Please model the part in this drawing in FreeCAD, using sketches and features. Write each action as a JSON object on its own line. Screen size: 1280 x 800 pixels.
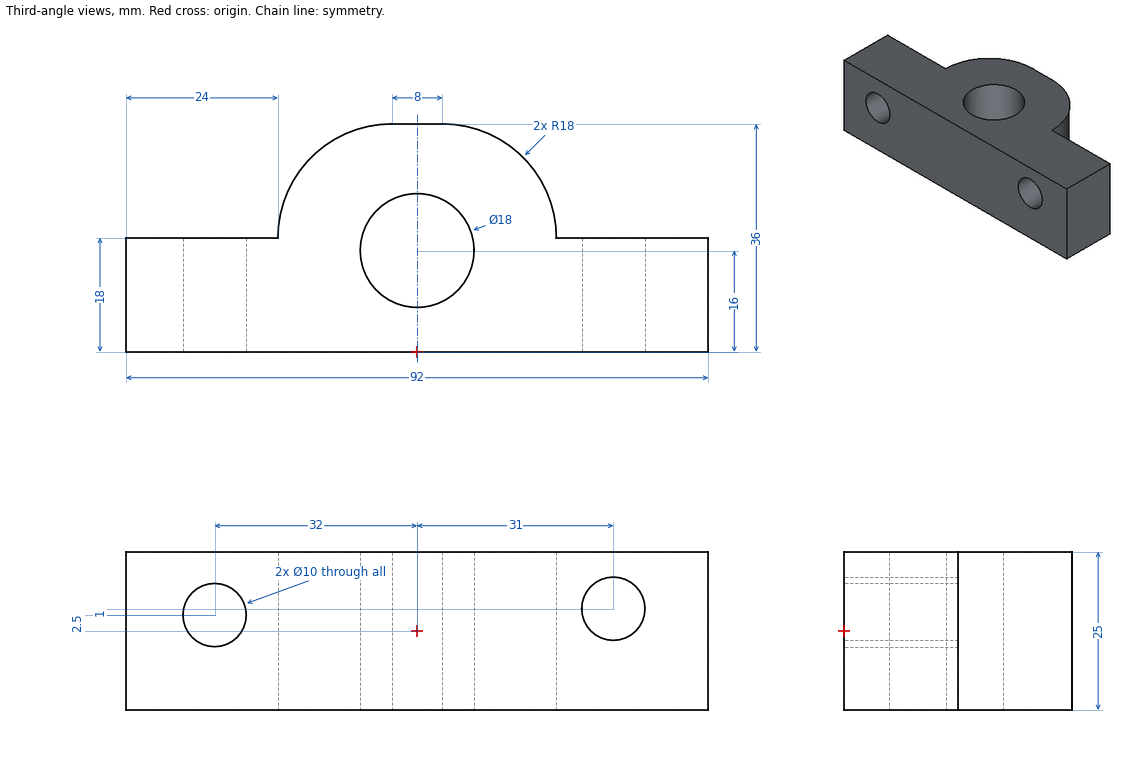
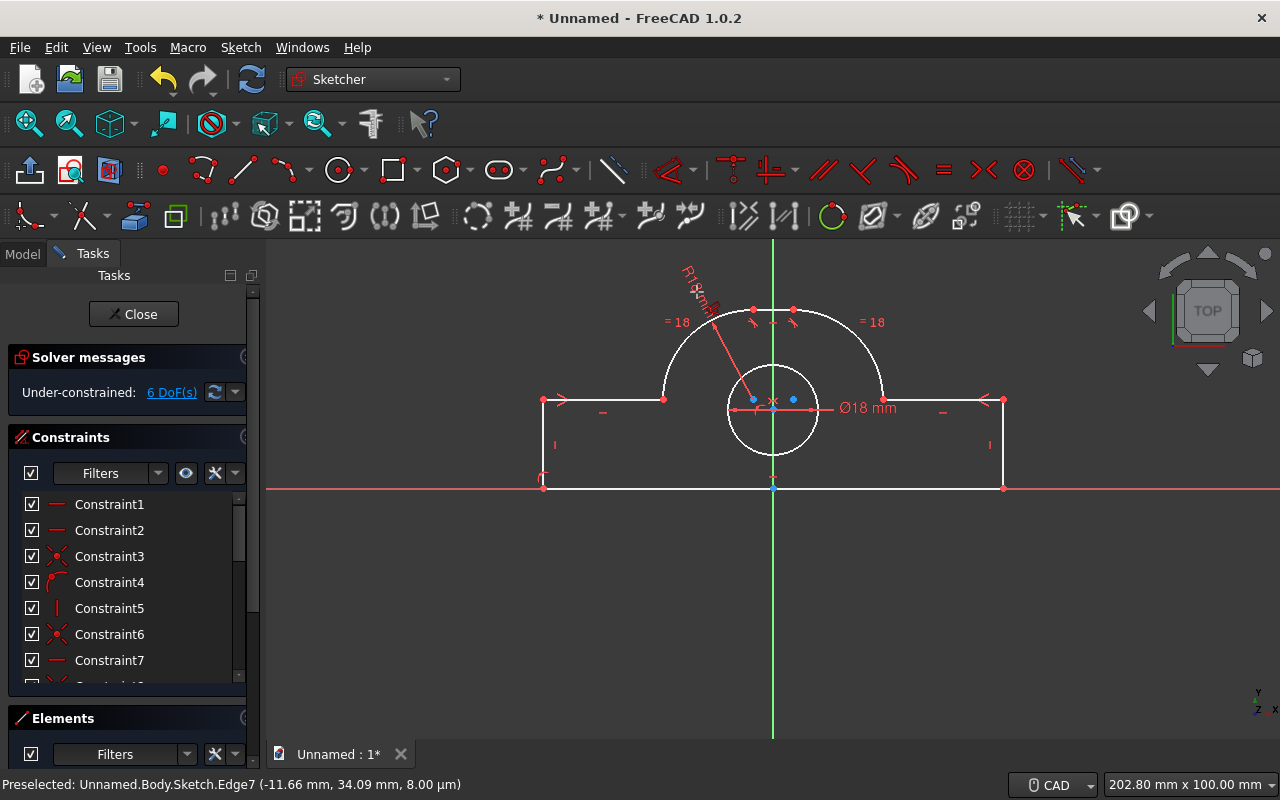
{"action": "left_click", "coordinate": [769, 310]}
{"action": "left_click", "coordinate": [787, 276]}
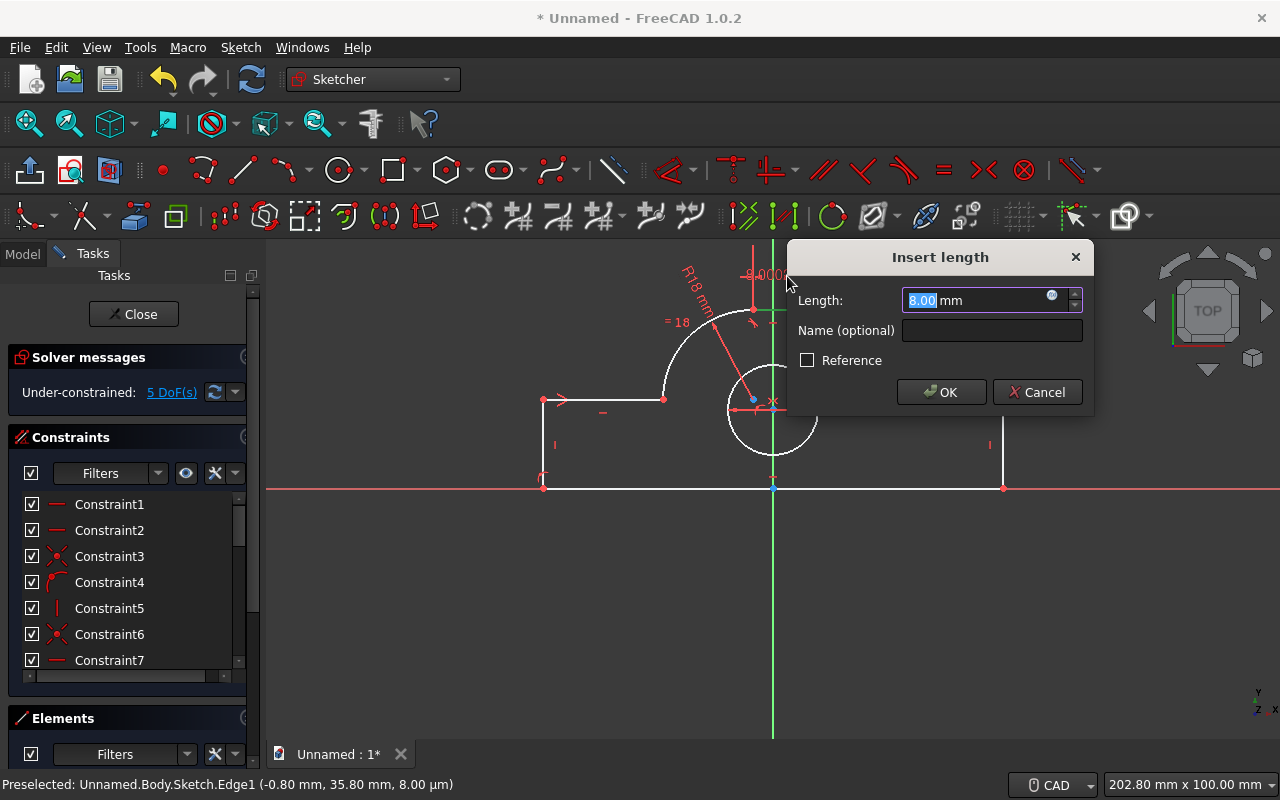
{"action": "type", "text": "8"}
{"action": "key", "text": "Return"}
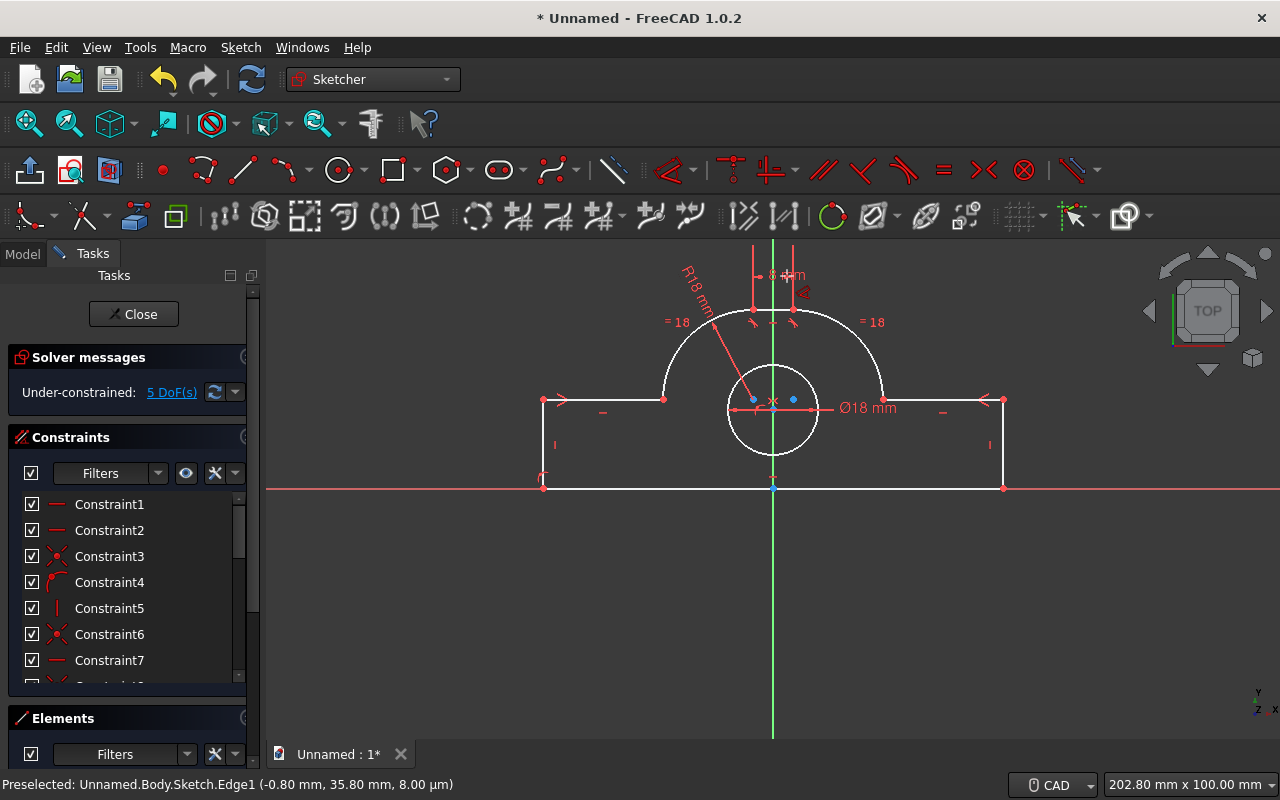
{"action": "left_click", "coordinate": [627, 400]}
{"action": "left_click", "coordinate": [603, 434]}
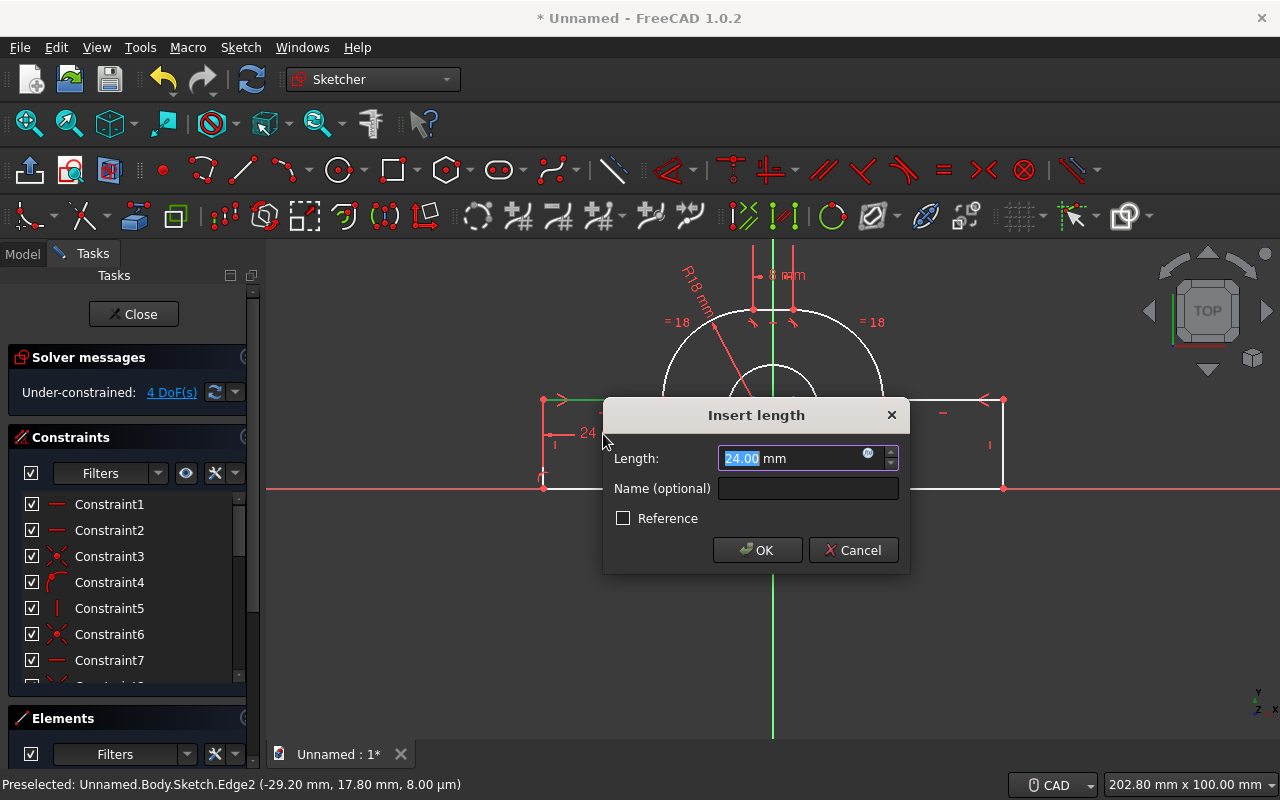
{"action": "type", "text": "24"}
{"action": "key", "text": "Return"}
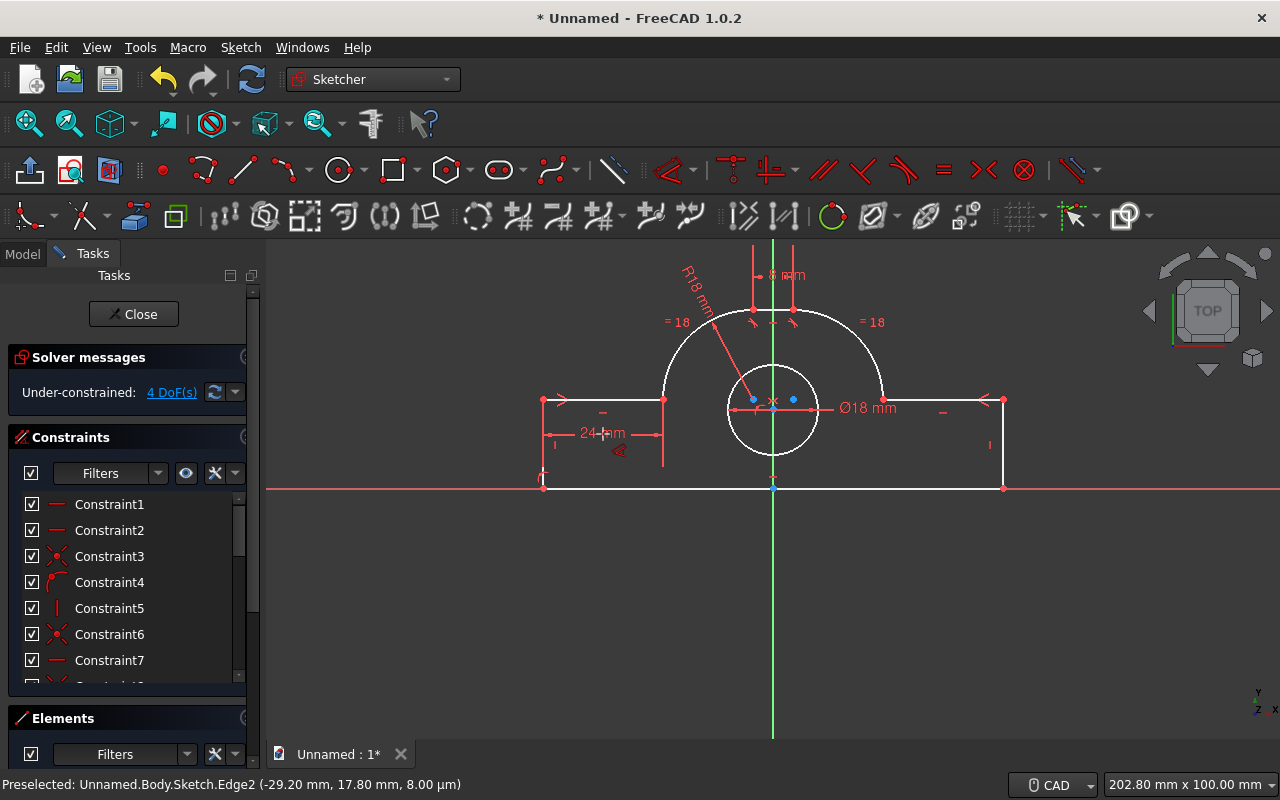
{"action": "left_click", "coordinate": [543, 427]}
{"action": "left_click", "coordinate": [509, 445]}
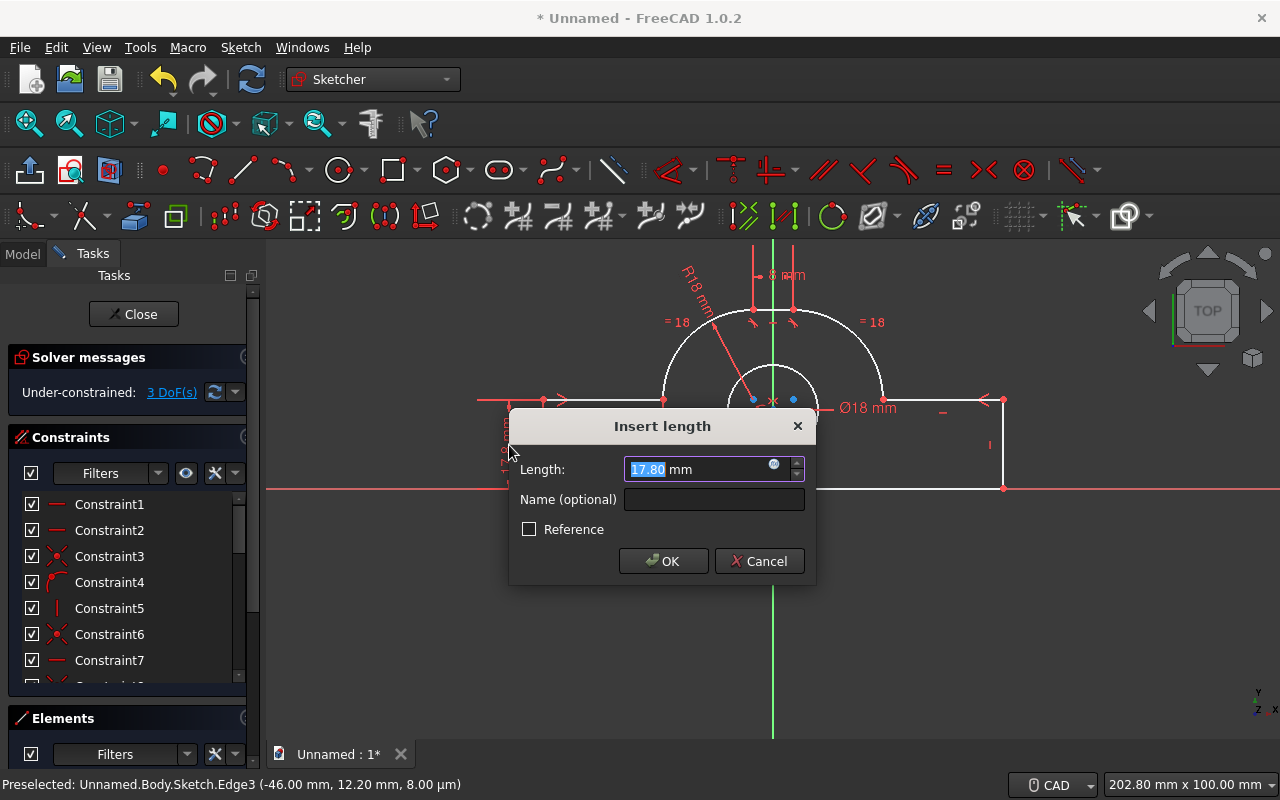
{"action": "type", "text": "18"}
{"action": "key", "text": "Return"}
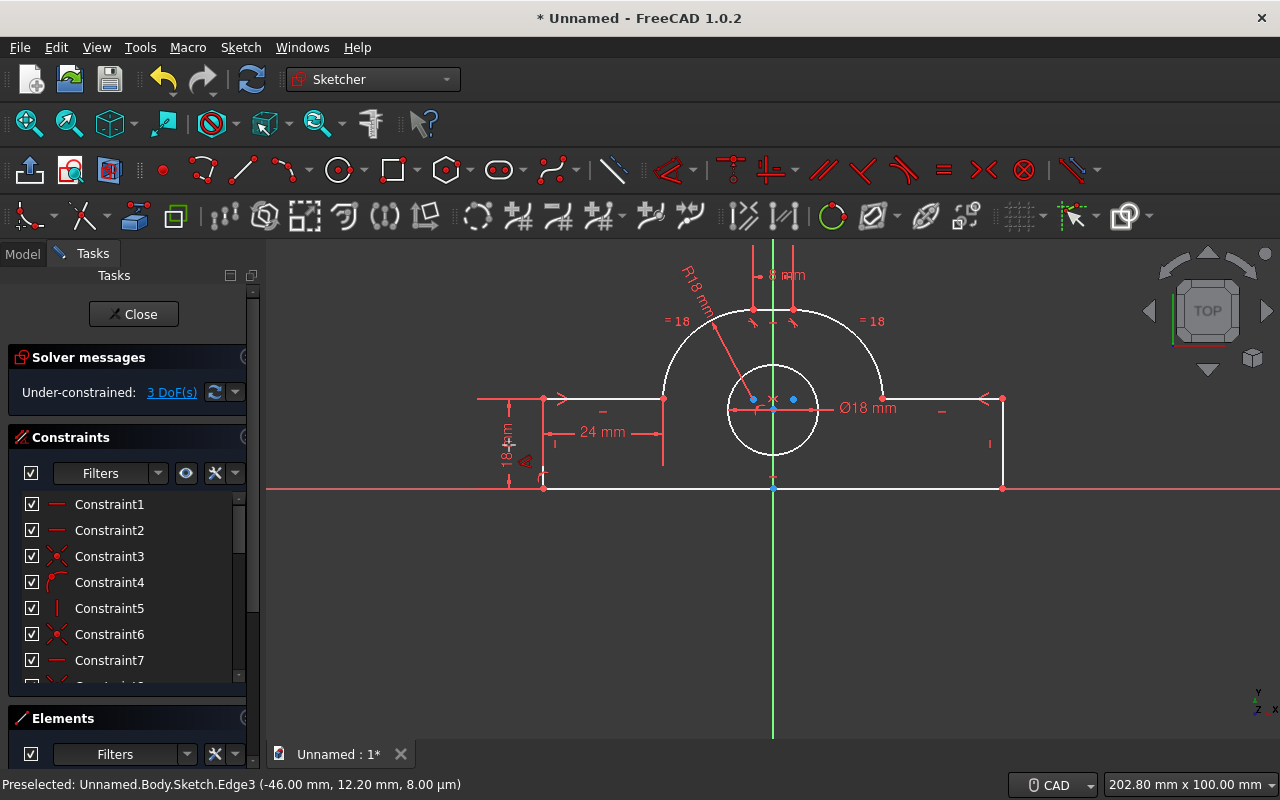
{"action": "left_click", "coordinate": [681, 489]}
{"action": "left_click", "coordinate": [667, 523]}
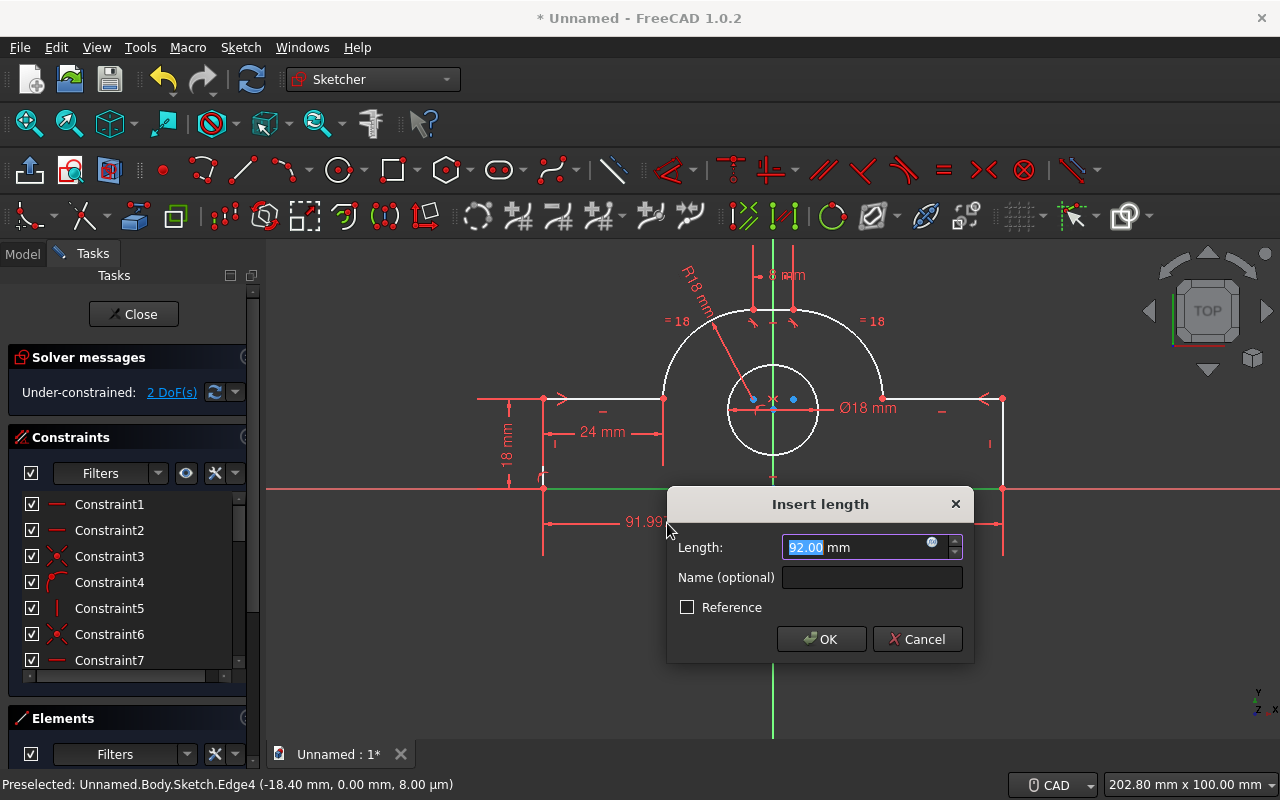
{"action": "type", "text": "92"}
{"action": "key", "text": "Return"}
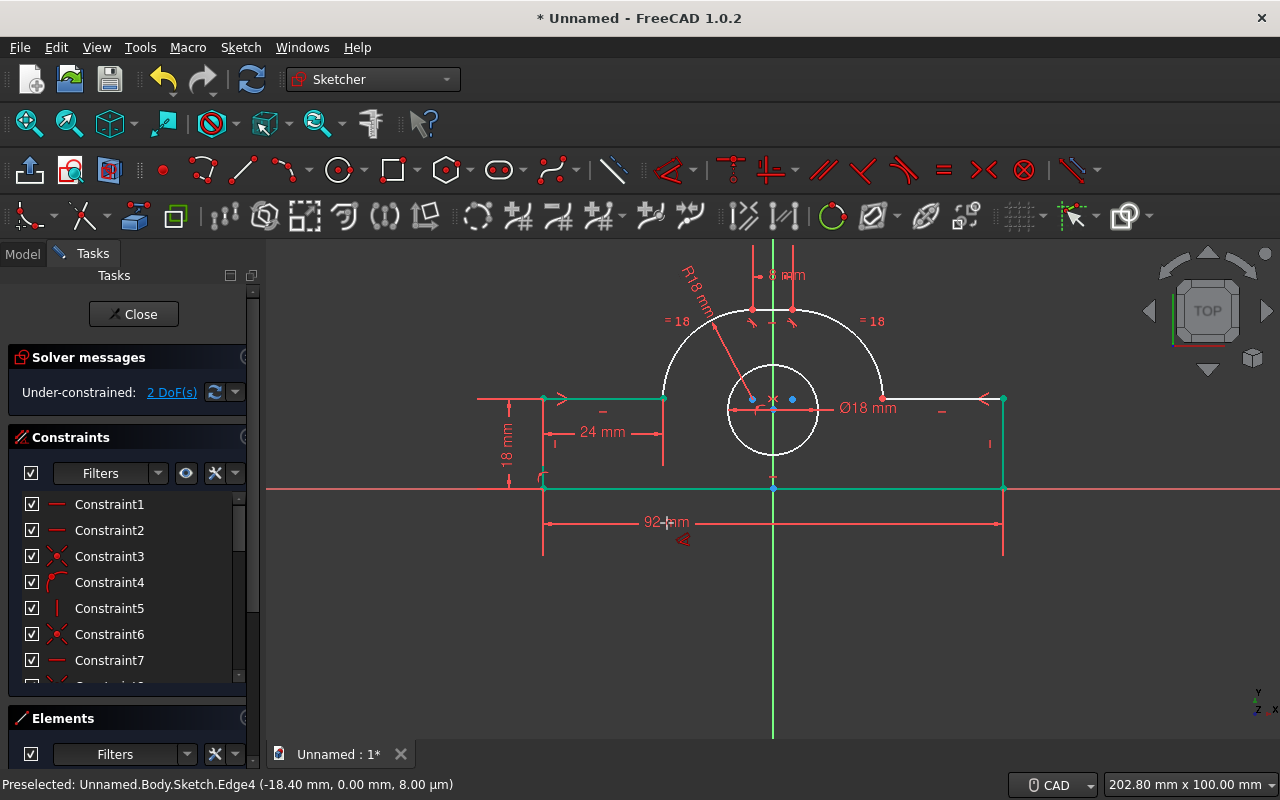
{"action": "left_click", "coordinate": [773, 410]}
{"action": "left_click", "coordinate": [807, 468]}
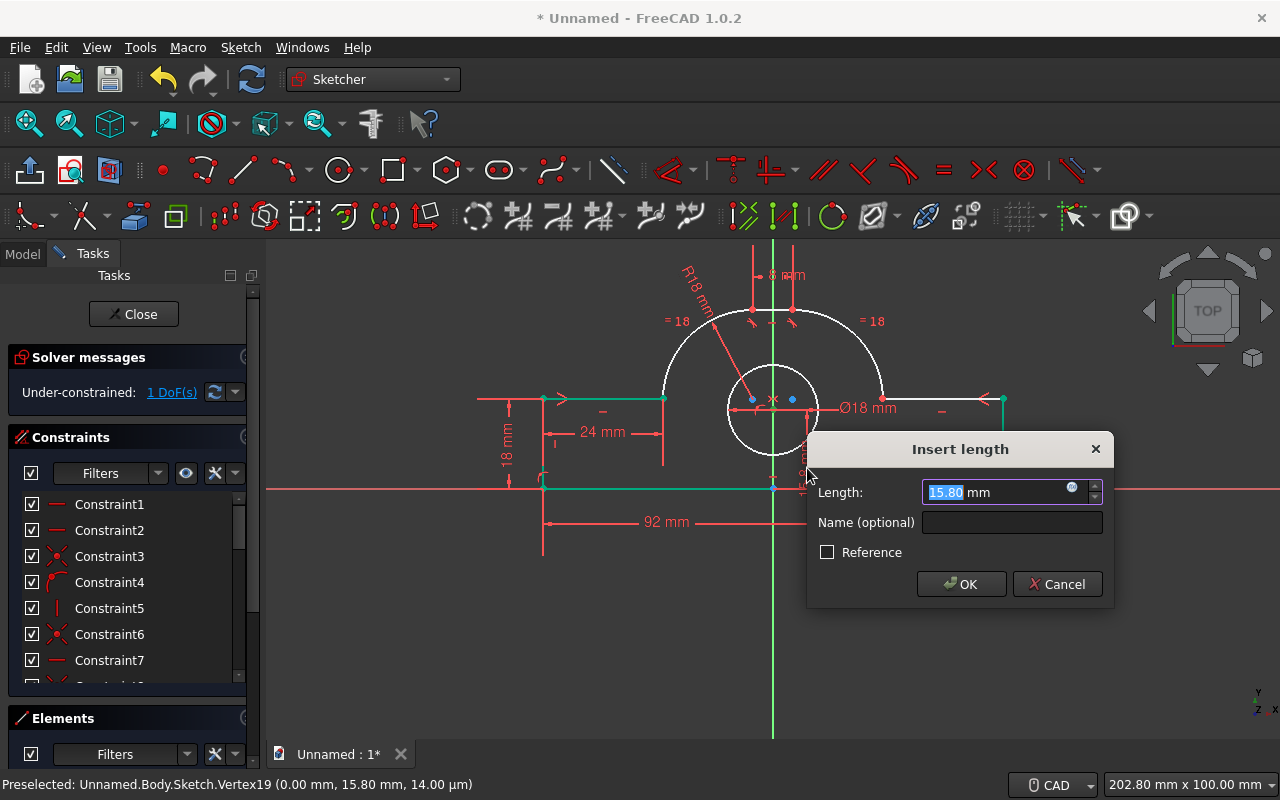
{"action": "type", "text": "16"}
{"action": "key", "text": "Return"}